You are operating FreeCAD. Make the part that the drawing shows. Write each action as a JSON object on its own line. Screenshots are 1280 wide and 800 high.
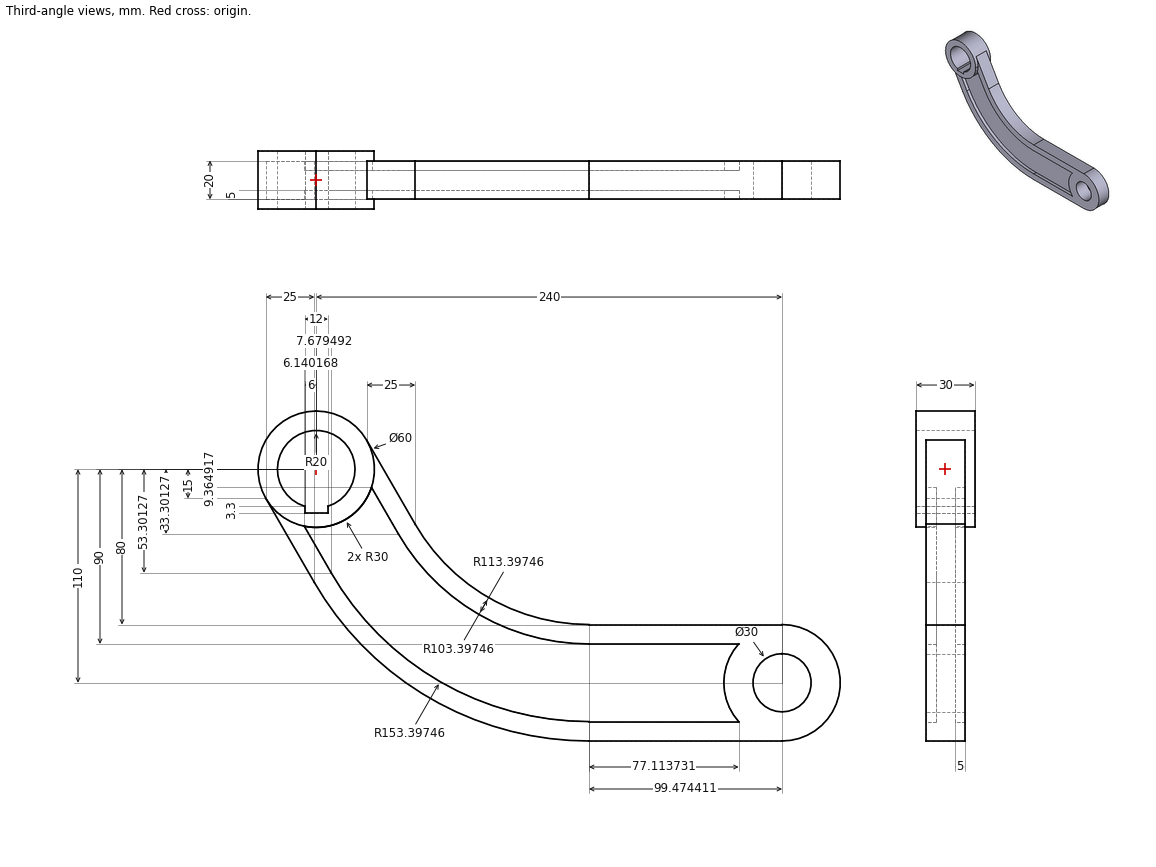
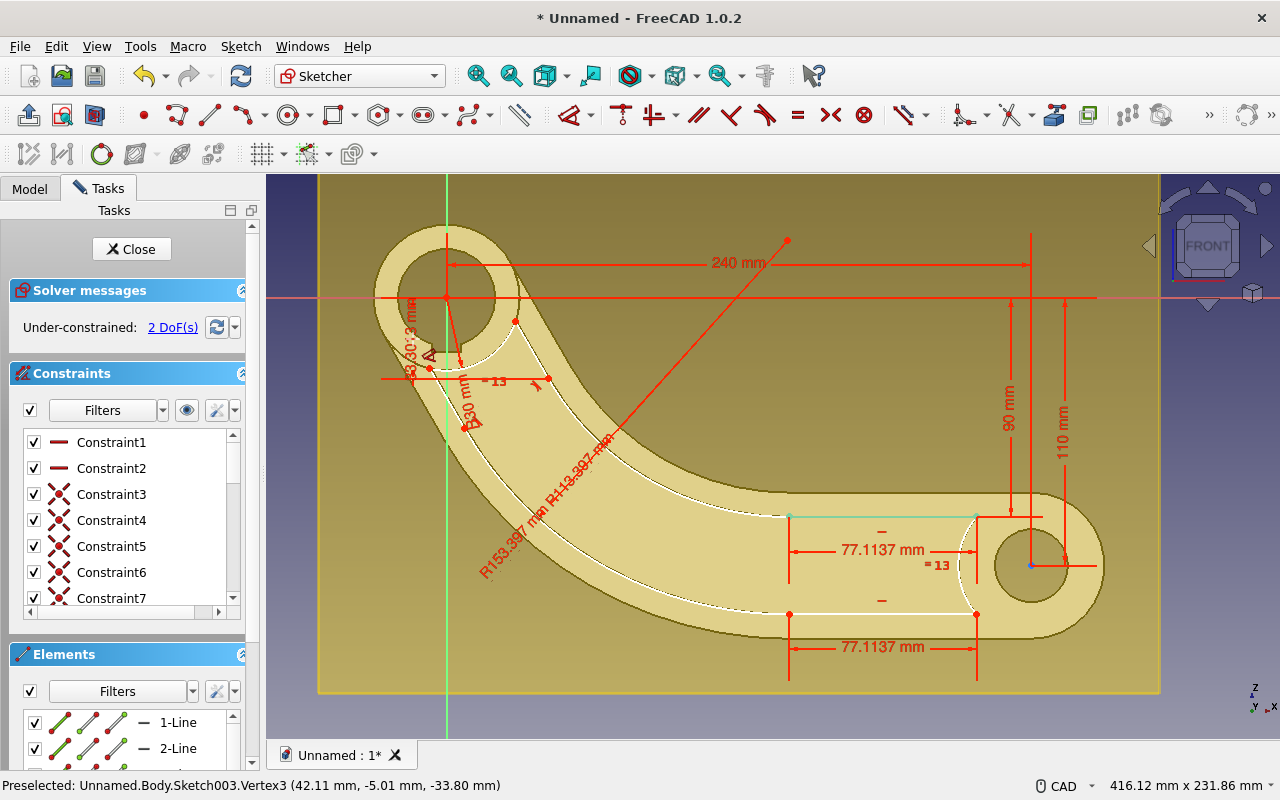
{"action": "scroll", "coordinate": [516, 322], "scroll_direction": "up", "scroll_amount": 3}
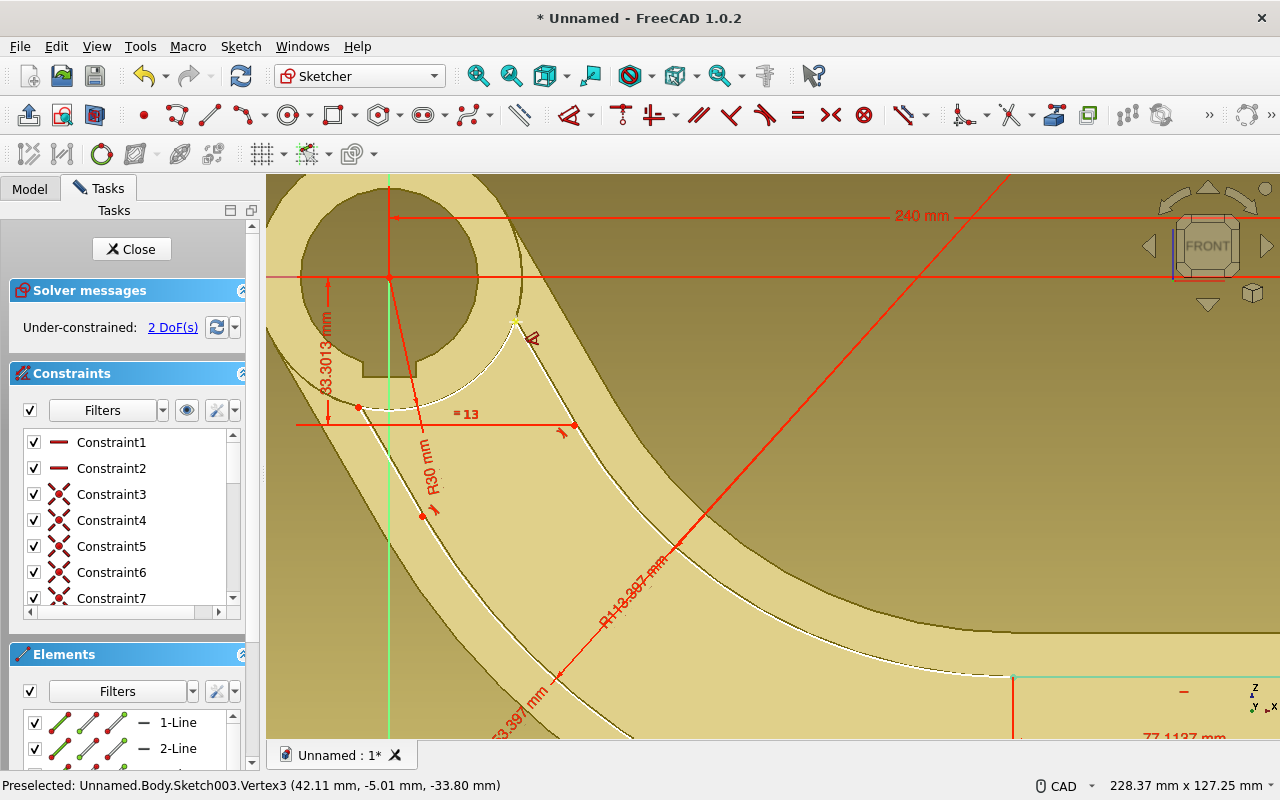
{"action": "left_click", "coordinate": [515, 321]}
{"action": "left_click", "coordinate": [355, 299]}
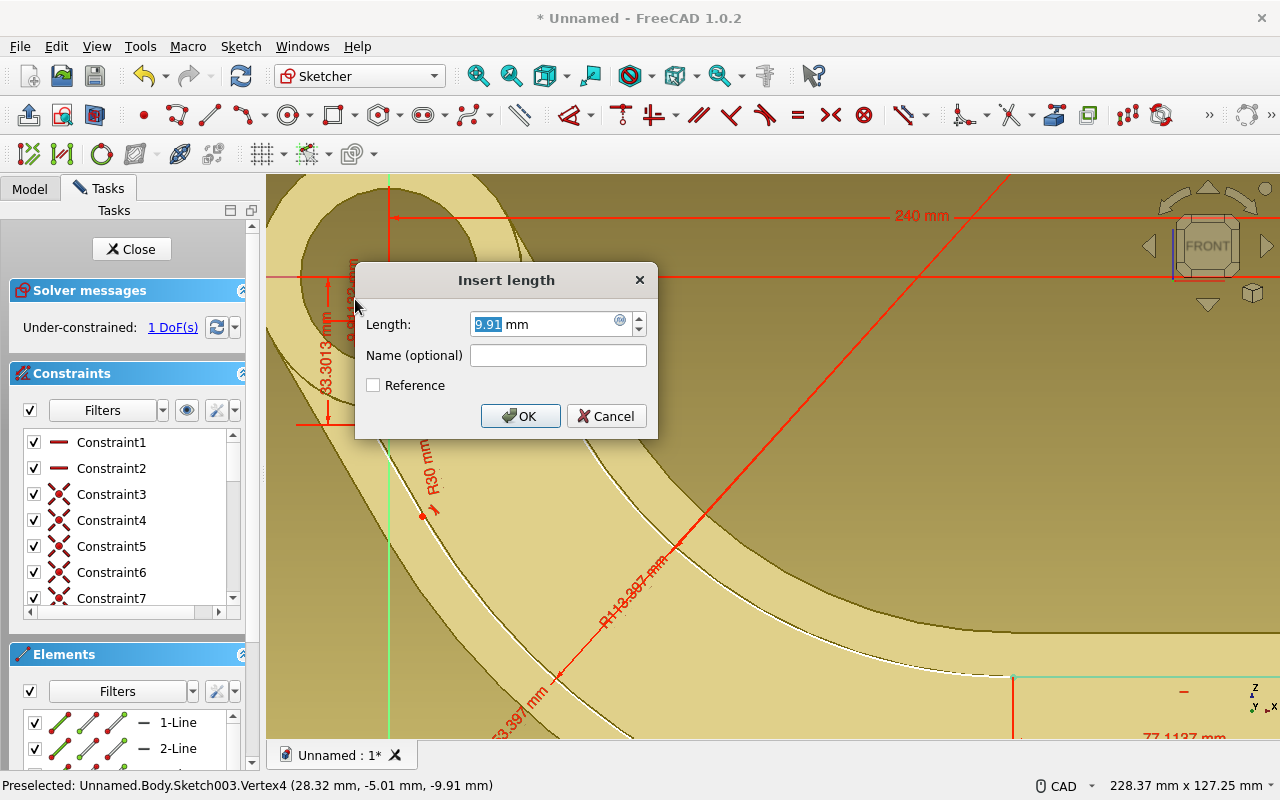
{"action": "type", "text": "9.364917"}
{"action": "key", "text": "Return"}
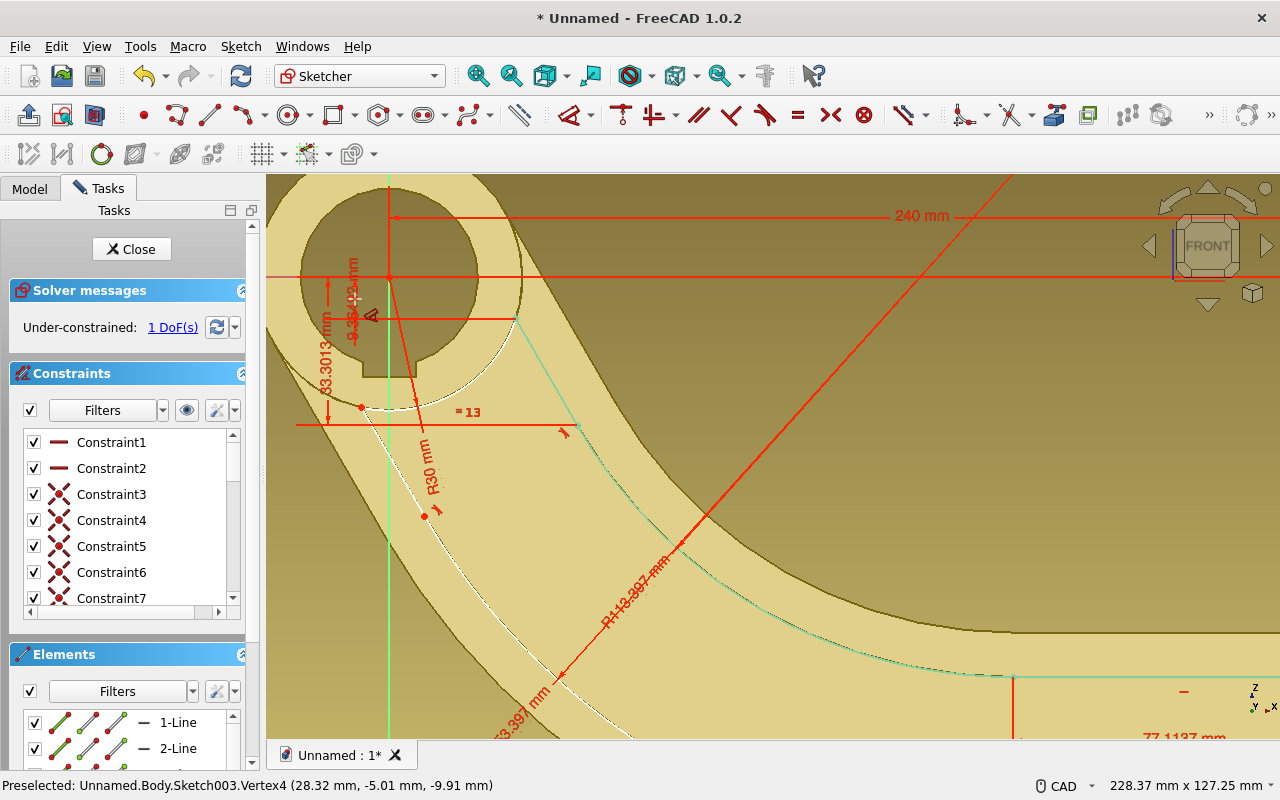
{"action": "scroll", "coordinate": [361, 408], "scroll_direction": "up", "scroll_amount": 2}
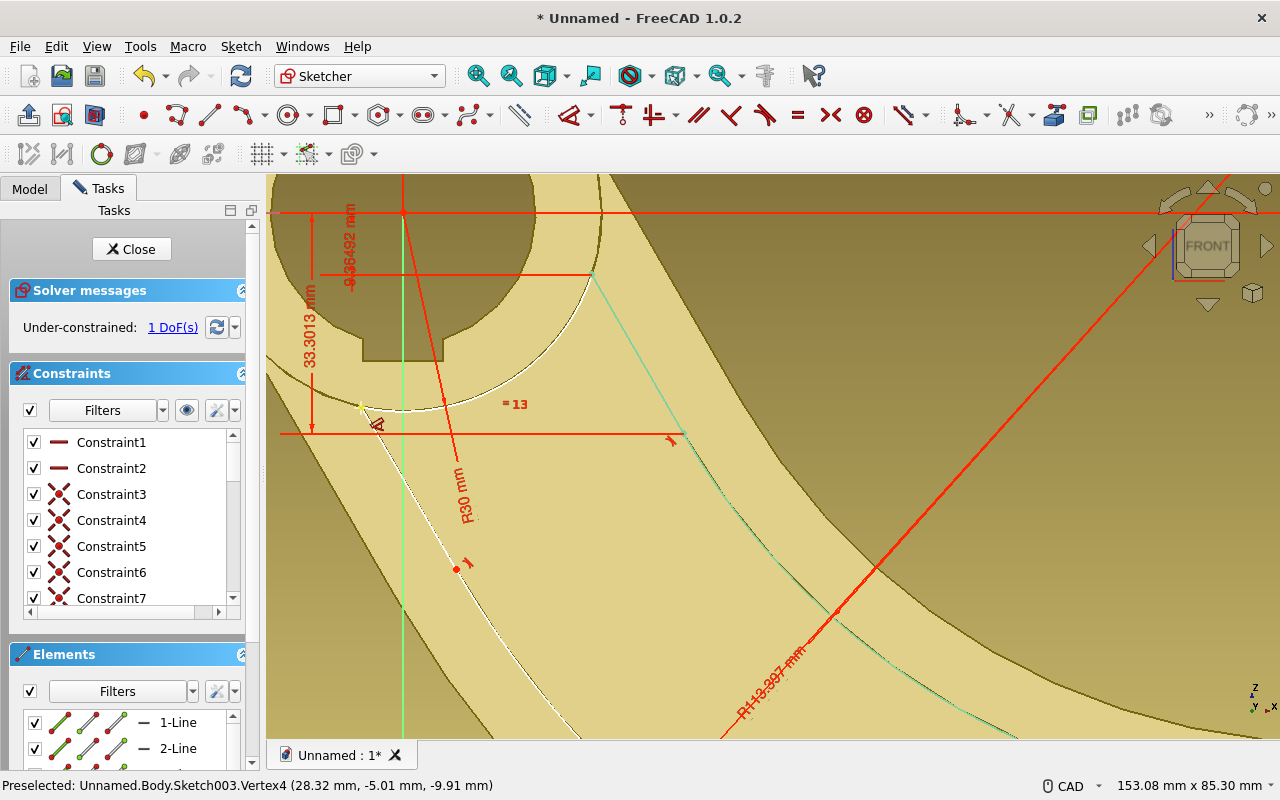
{"action": "left_click", "coordinate": [361, 407]}
{"action": "left_click", "coordinate": [373, 465]}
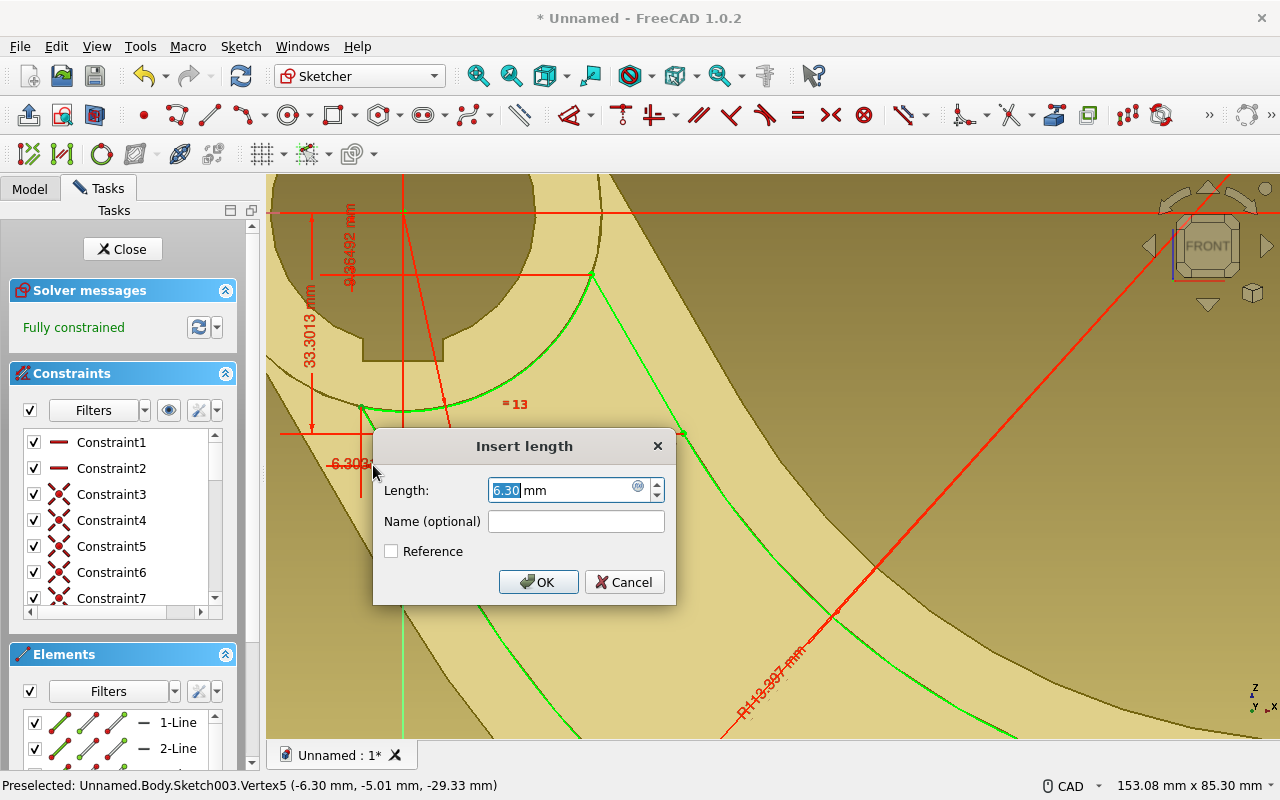
{"action": "type", "text": "6.140168"}
{"action": "key", "text": "Return"}
{"action": "key", "text": "Escape"}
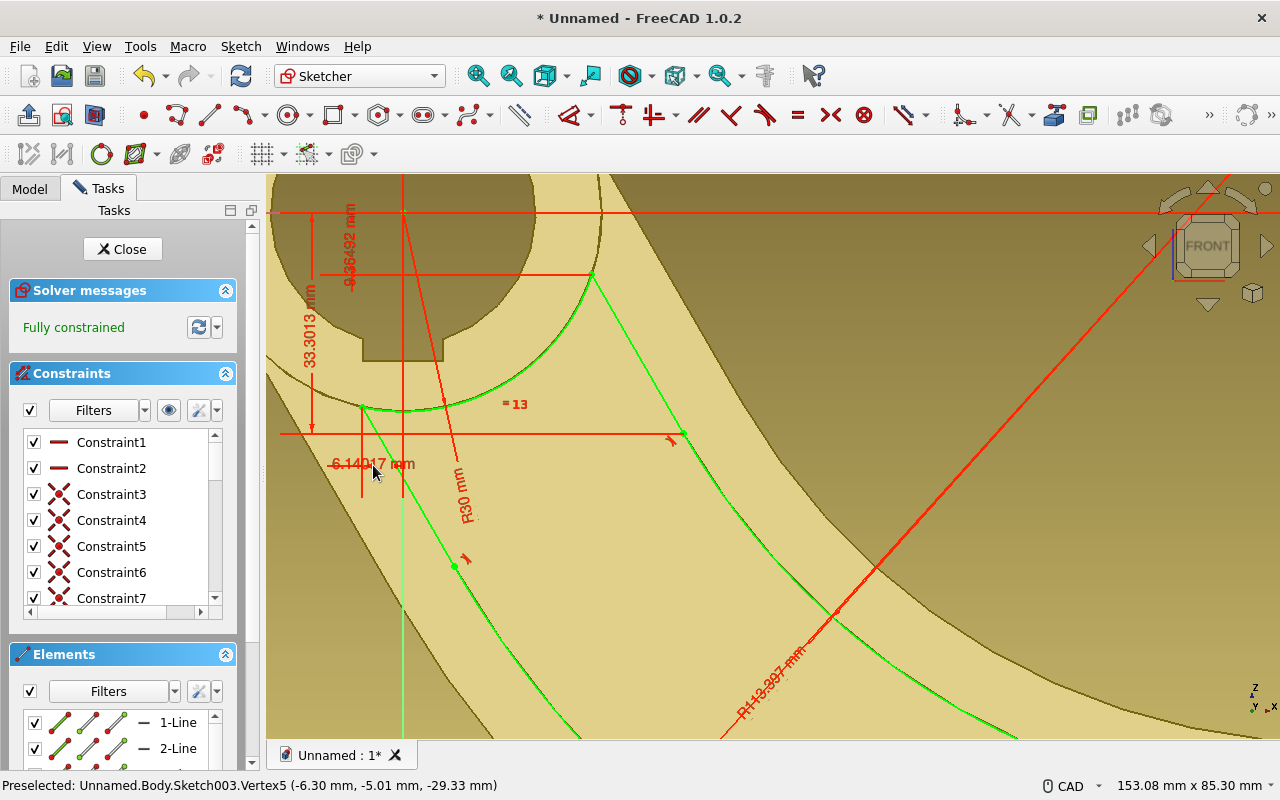
{"action": "left_click", "coordinate": [123, 249]}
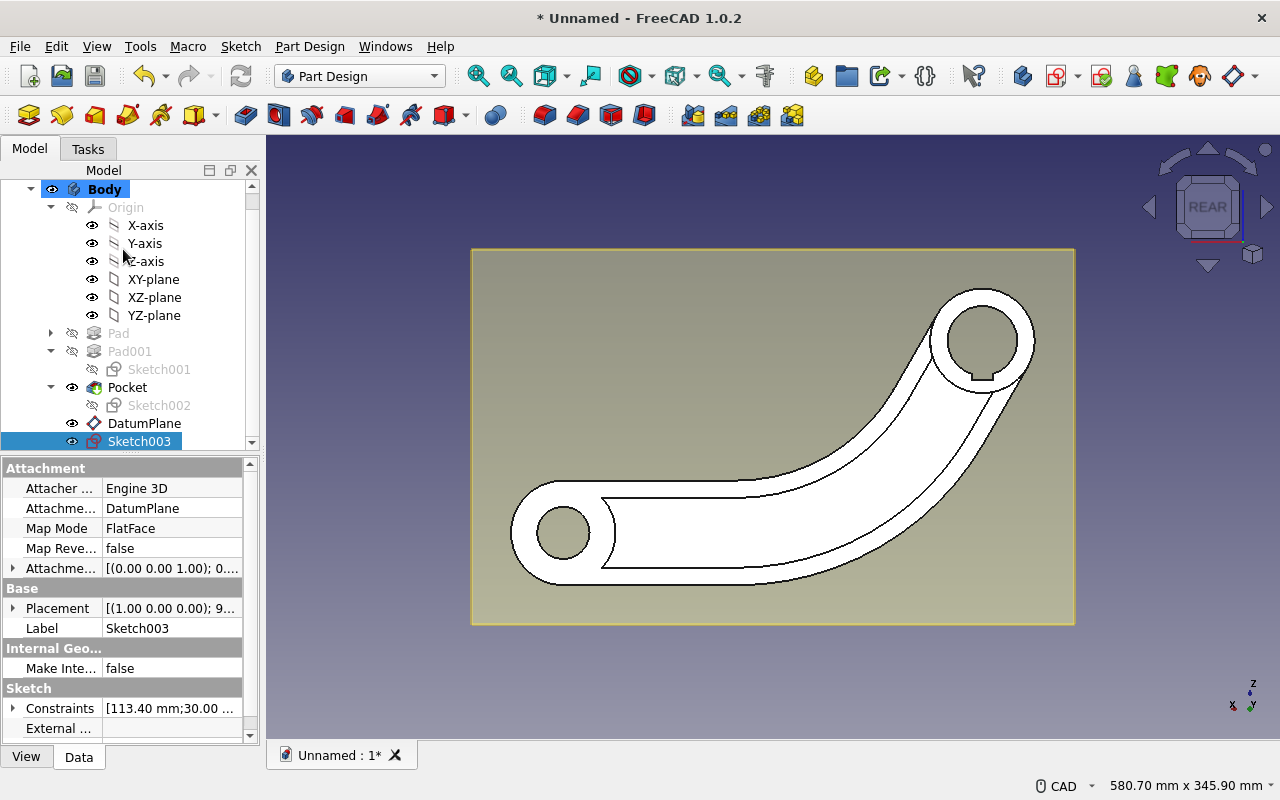
{"action": "left_click", "coordinate": [246, 116]}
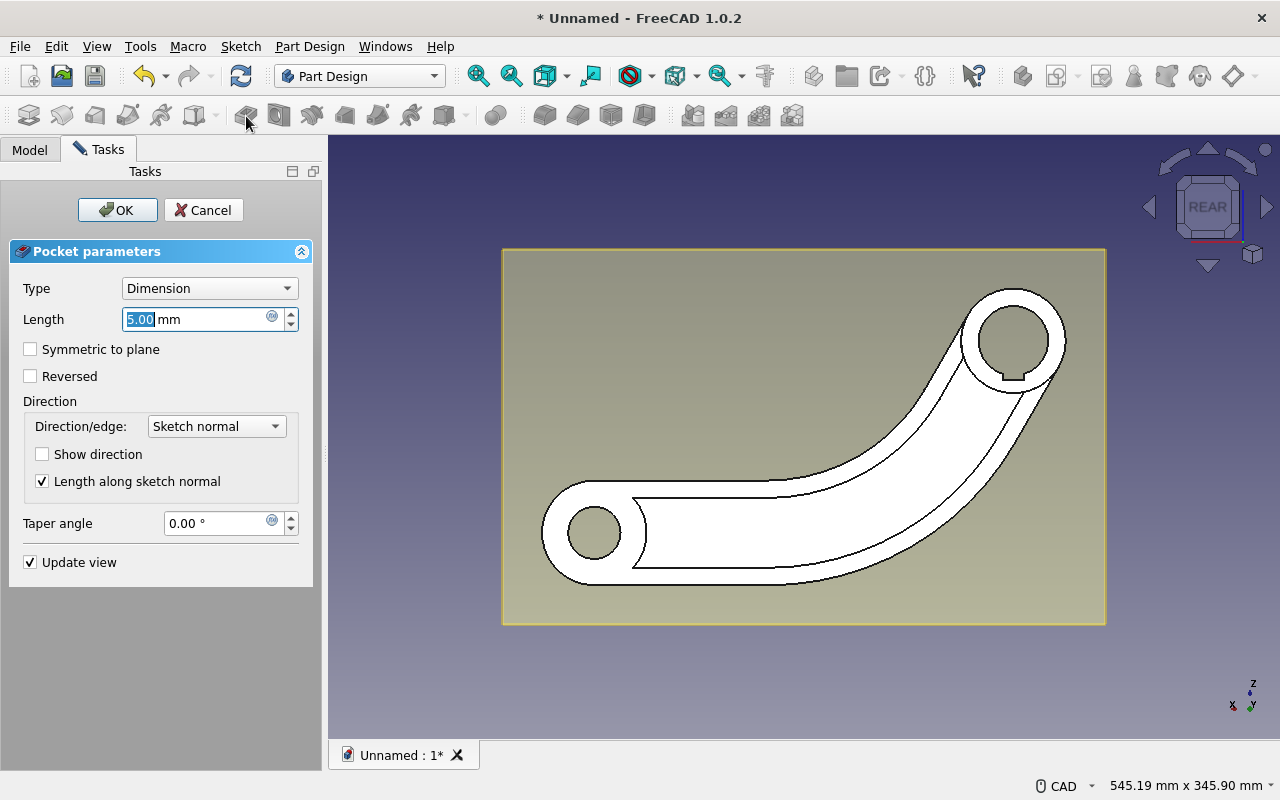
{"action": "type", "text": "5"}
{"action": "key", "text": "Tab"}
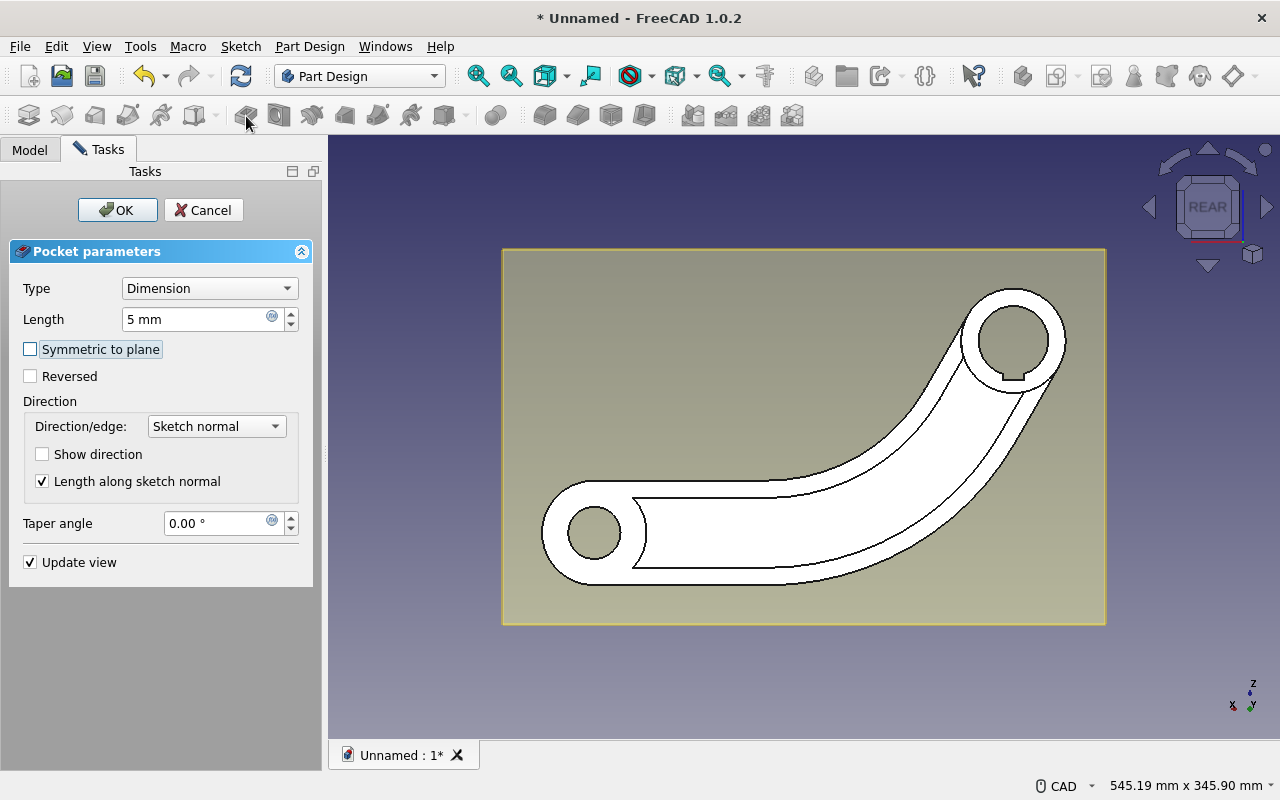
{"action": "left_click", "coordinate": [31, 376]}